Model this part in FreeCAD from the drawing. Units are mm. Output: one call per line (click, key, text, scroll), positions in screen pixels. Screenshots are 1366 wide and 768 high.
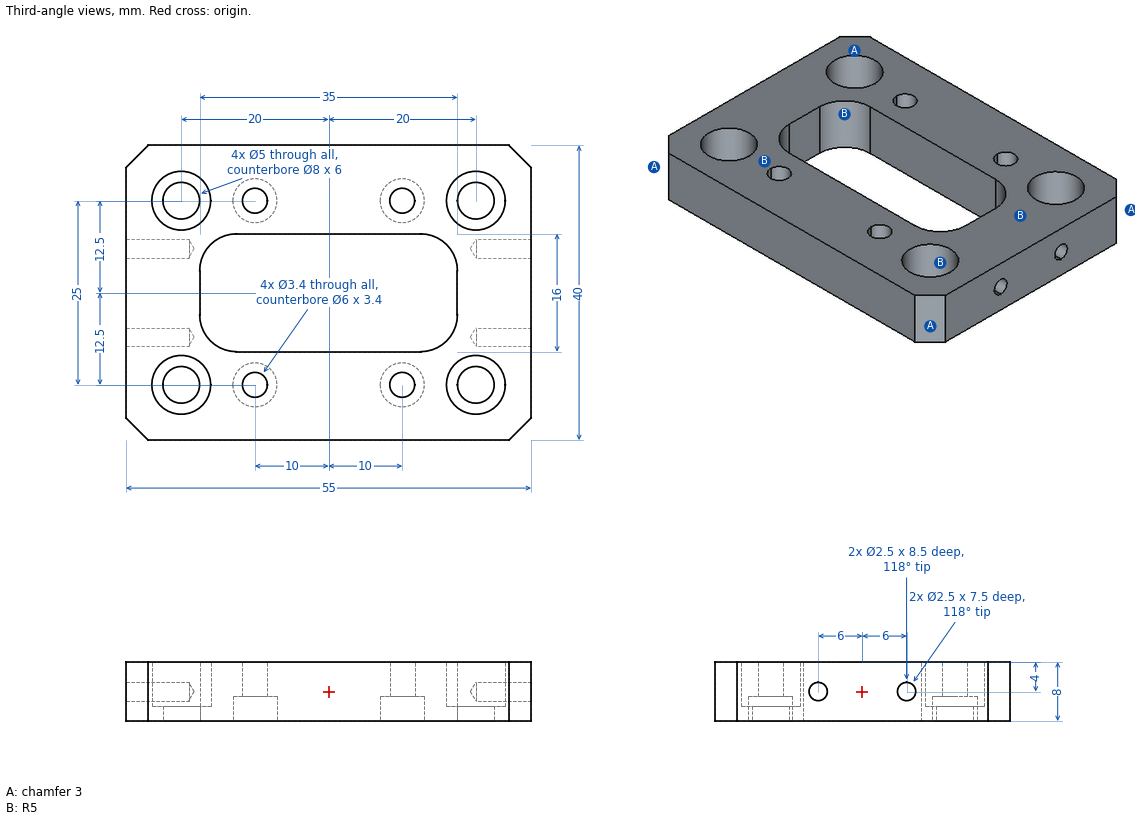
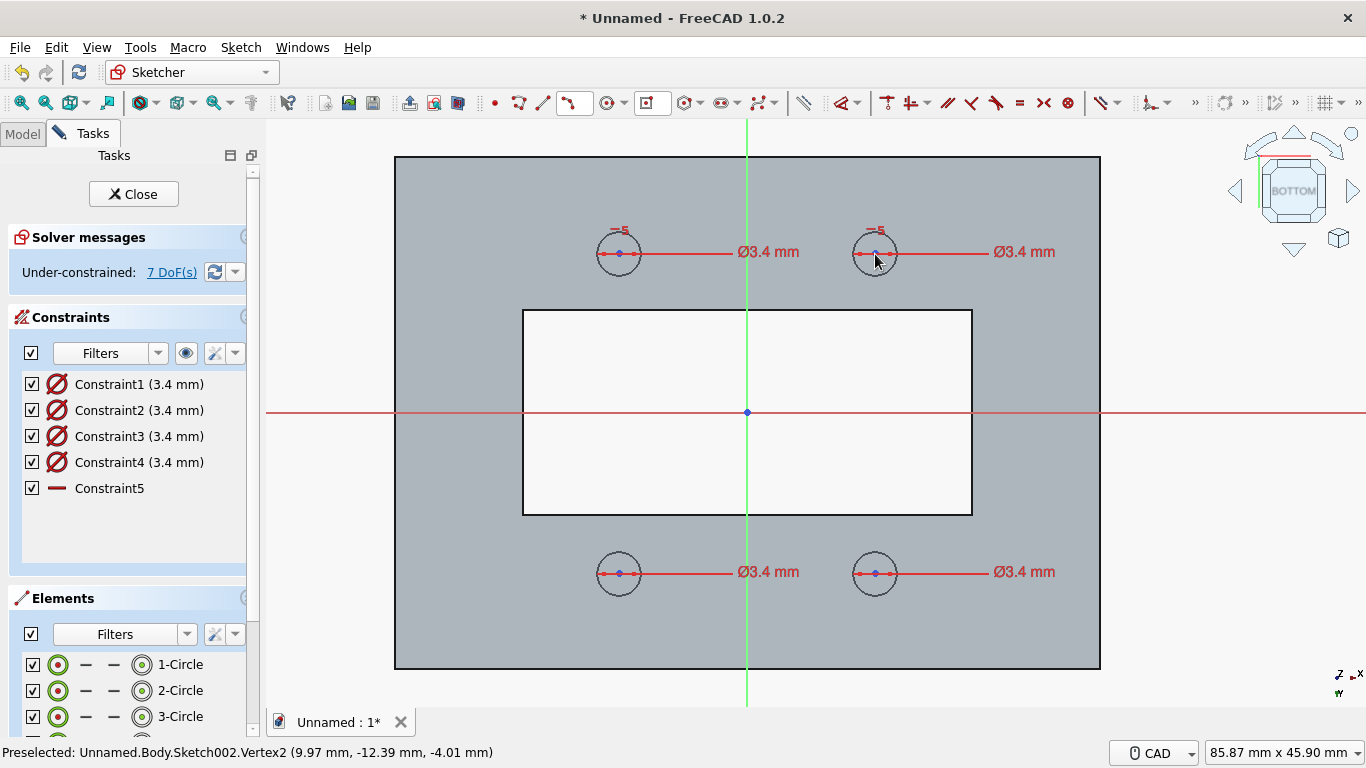
click(619, 254)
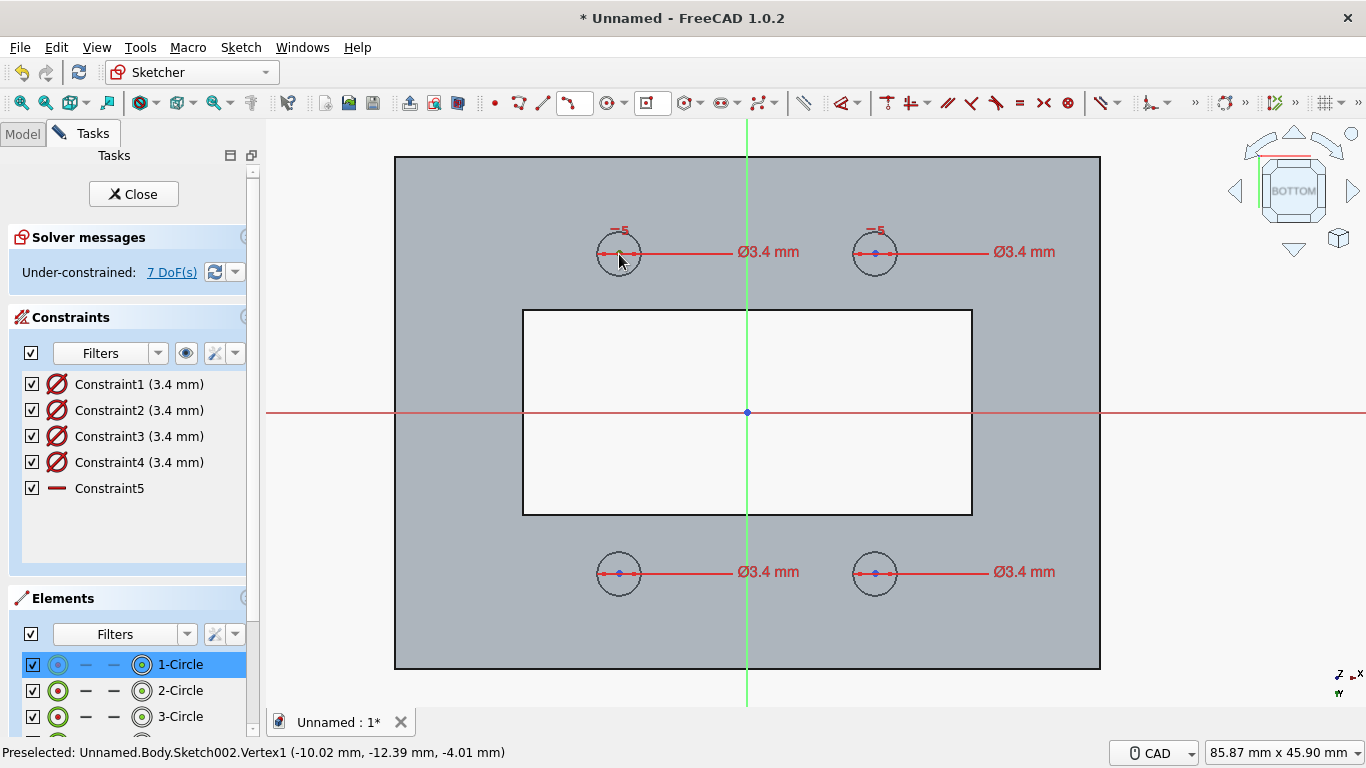
click(619, 574)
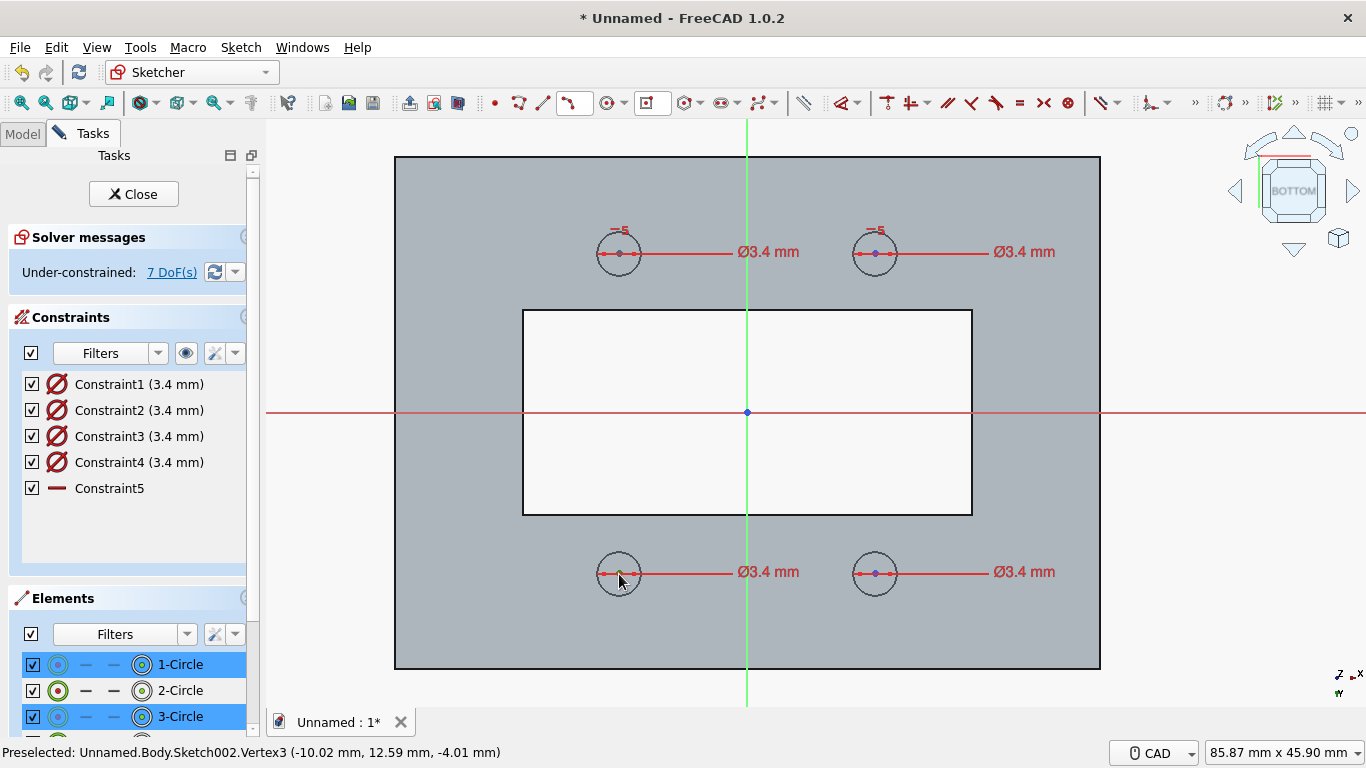
key(v)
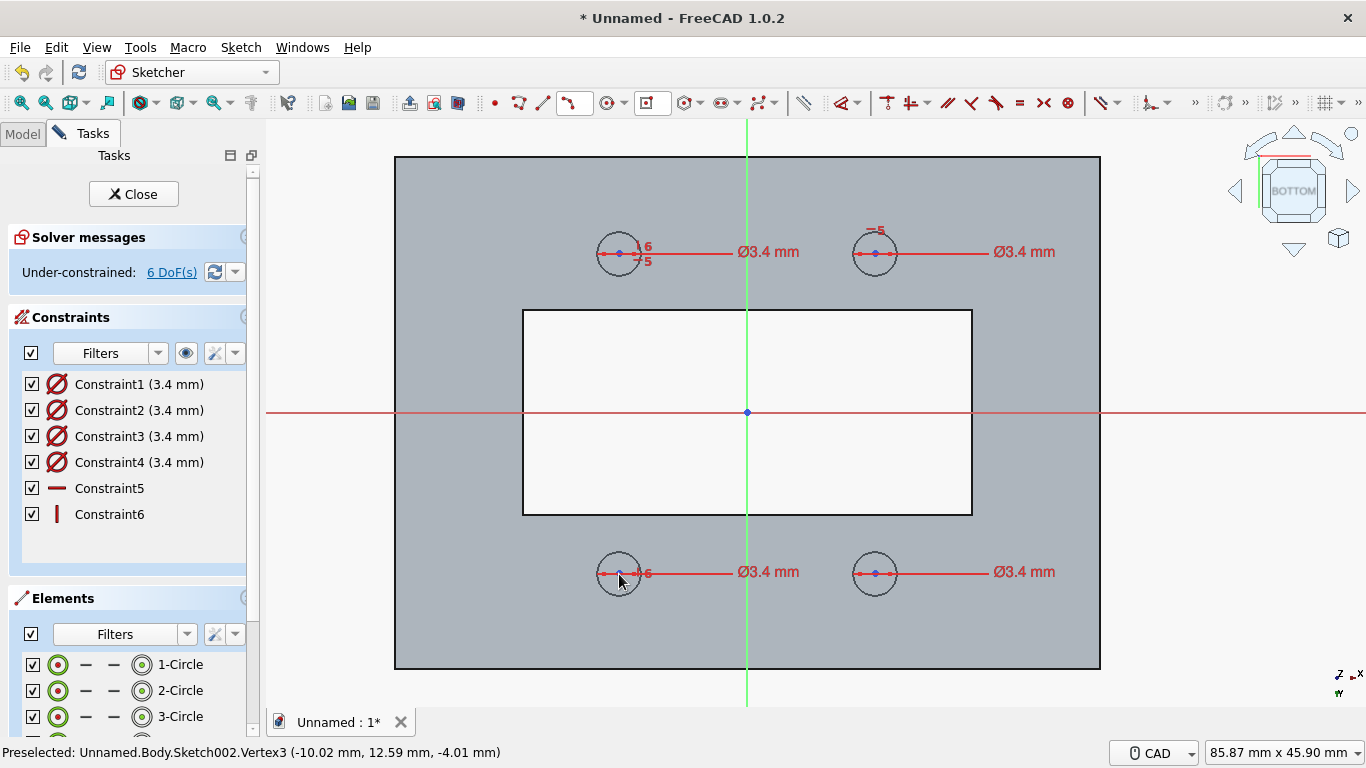
click(875, 254)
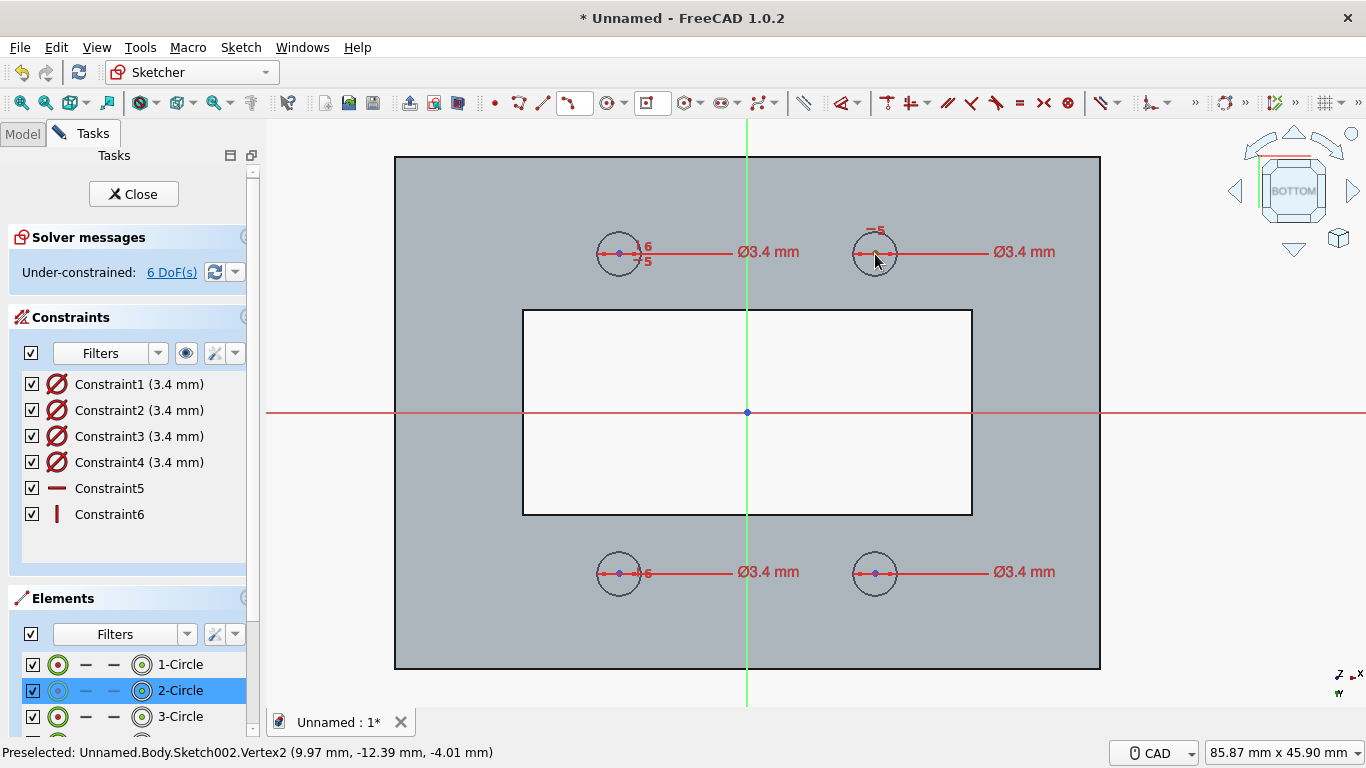
click(875, 574)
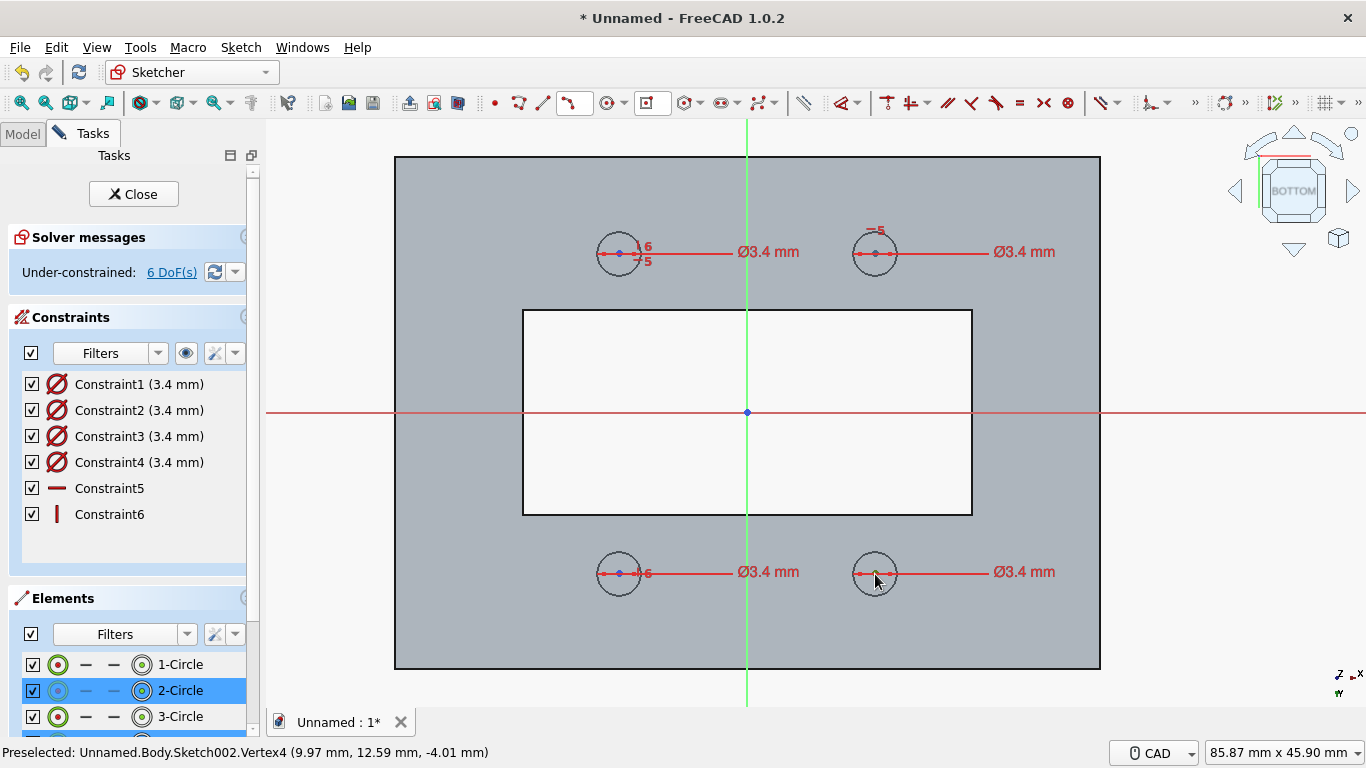
key(v)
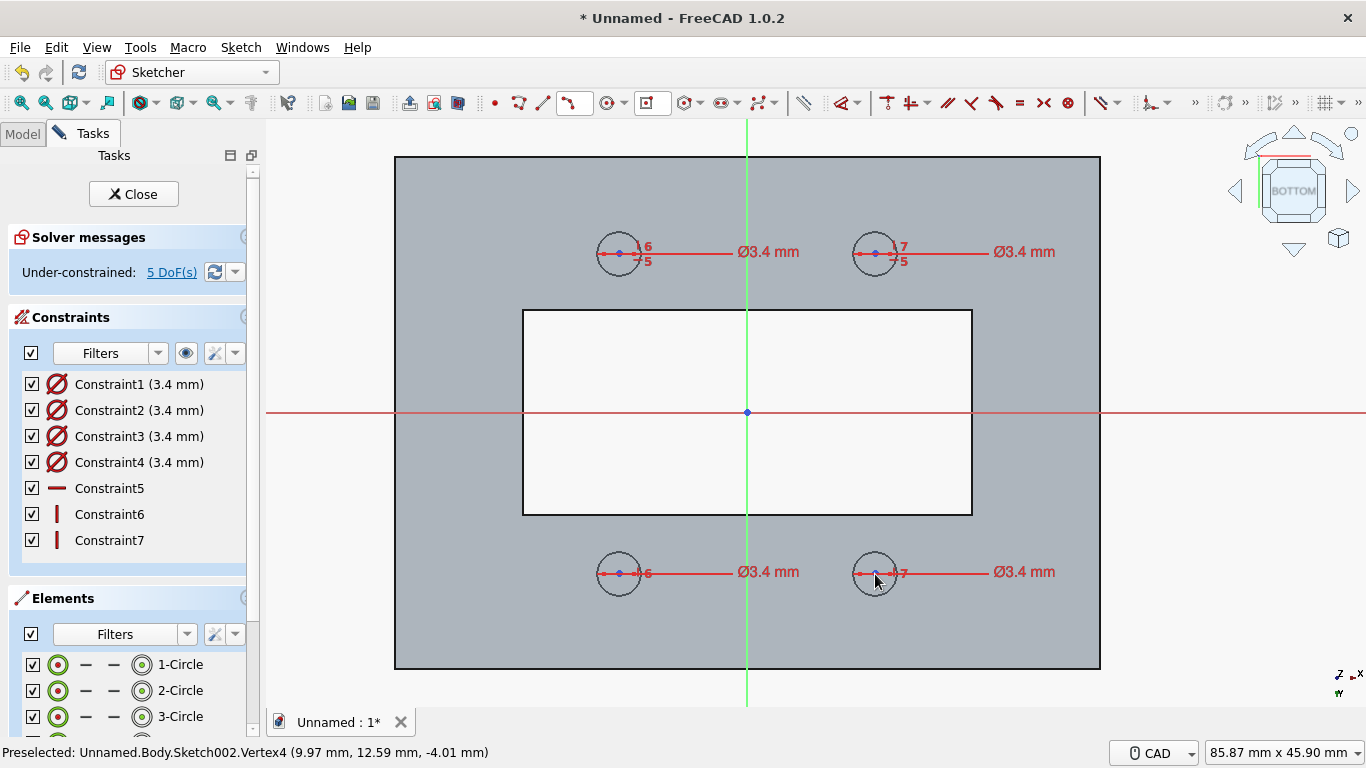
click(619, 574)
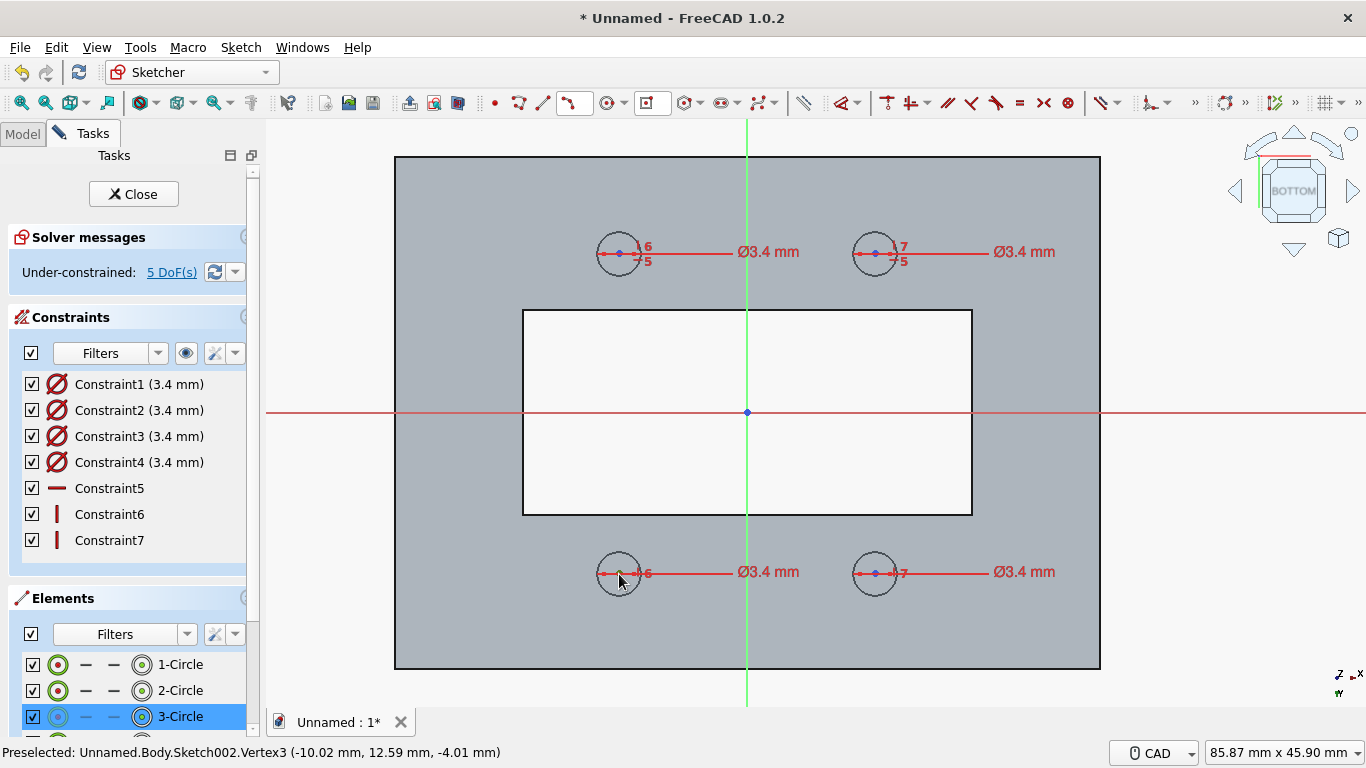
click(875, 574)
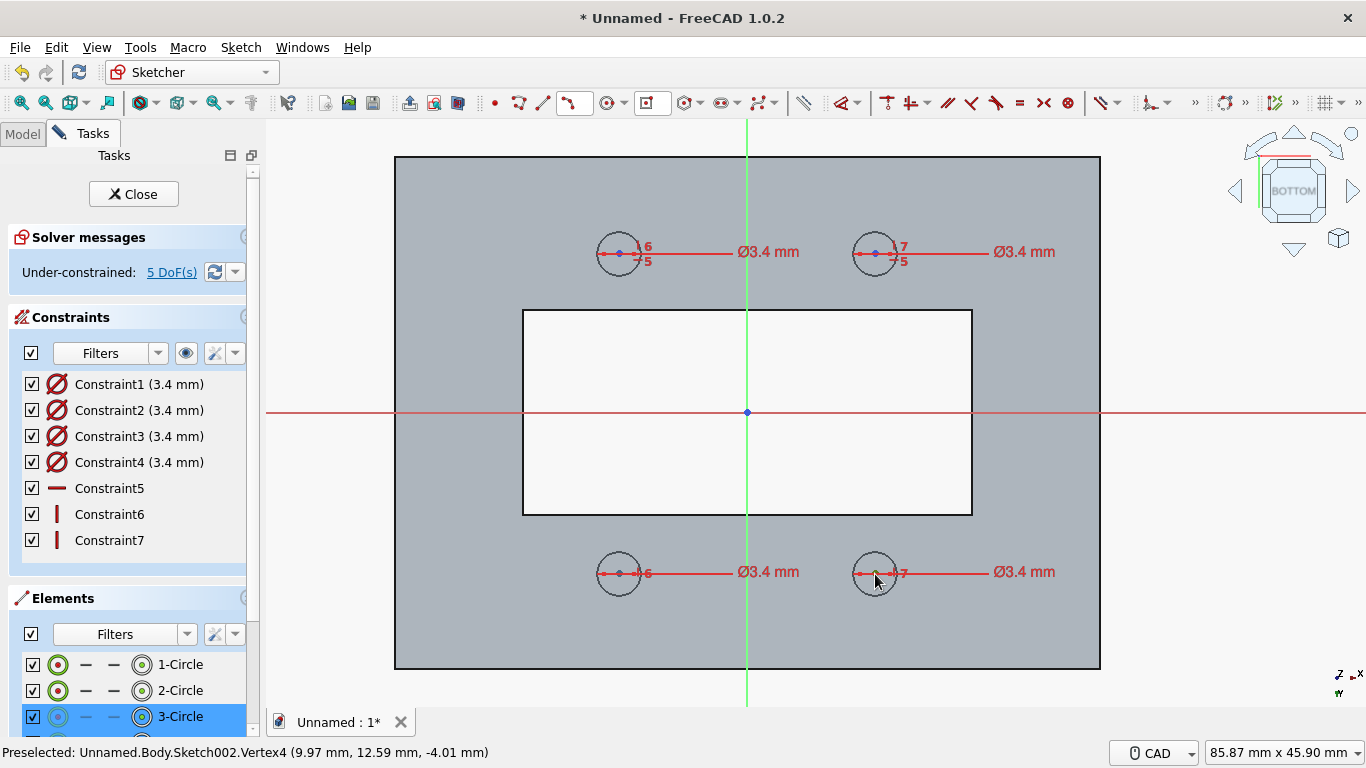
key(h)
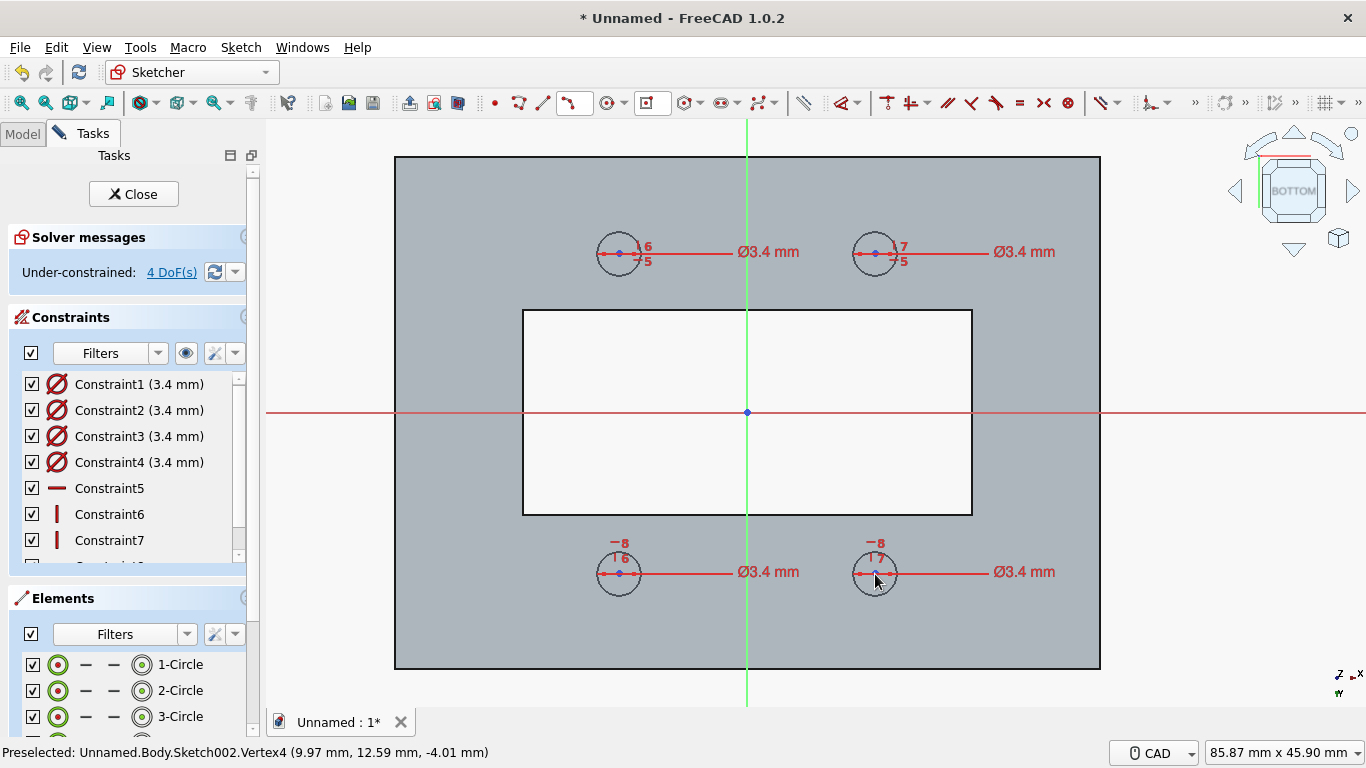
click(619, 254)